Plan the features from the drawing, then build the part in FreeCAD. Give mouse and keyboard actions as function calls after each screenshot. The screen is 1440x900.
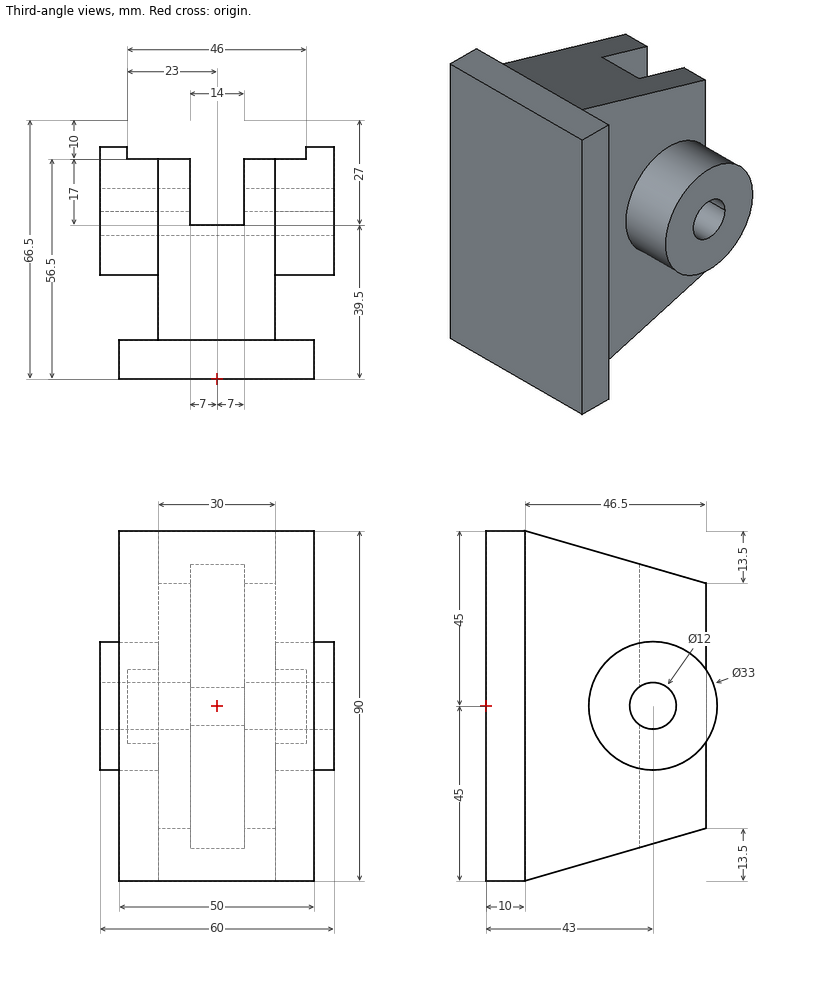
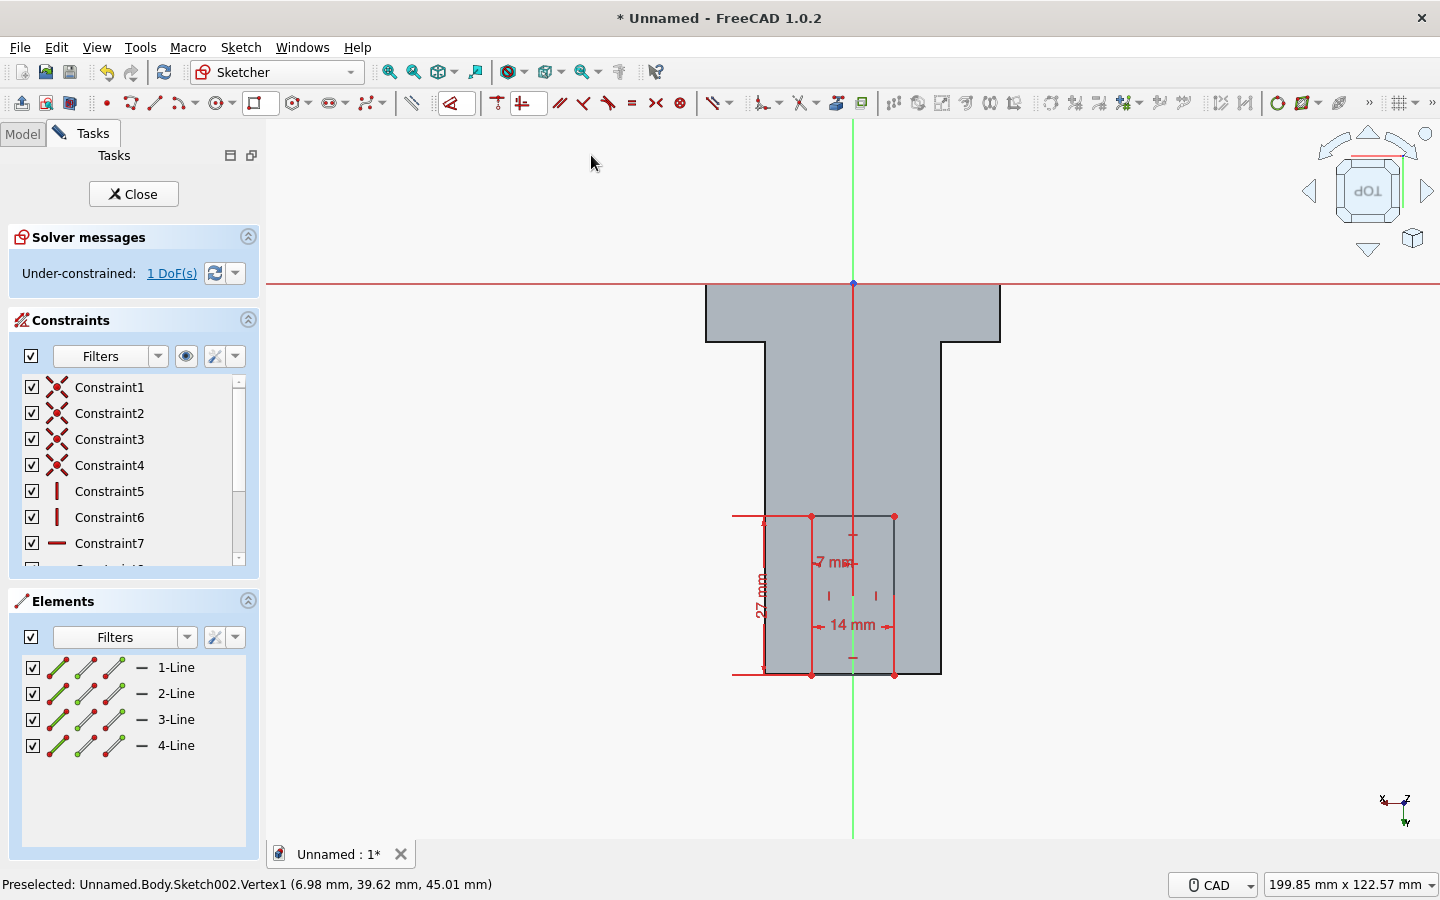
click(812, 516)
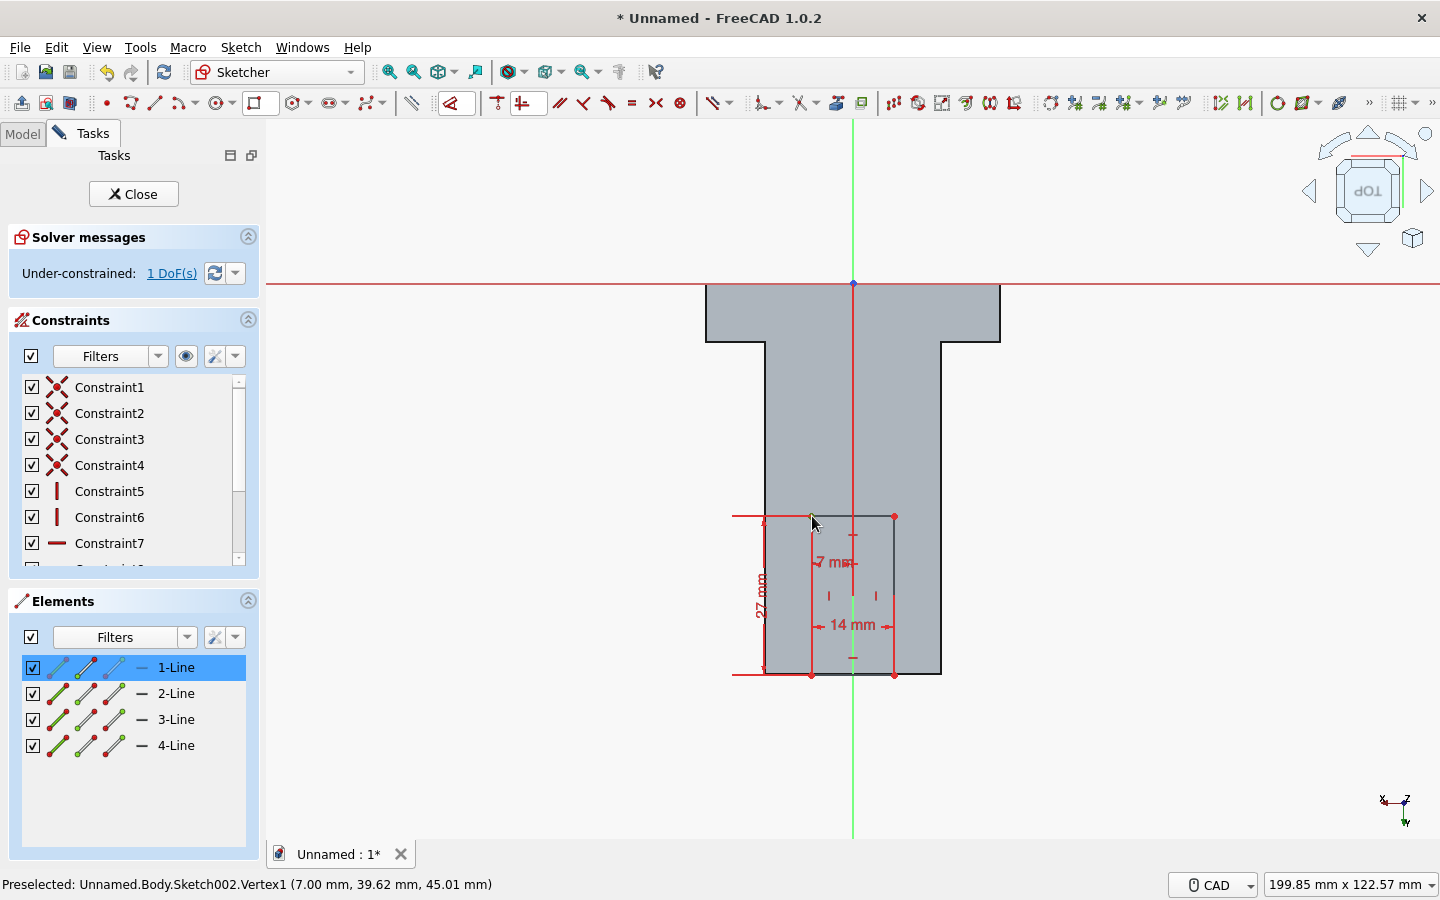
key(i)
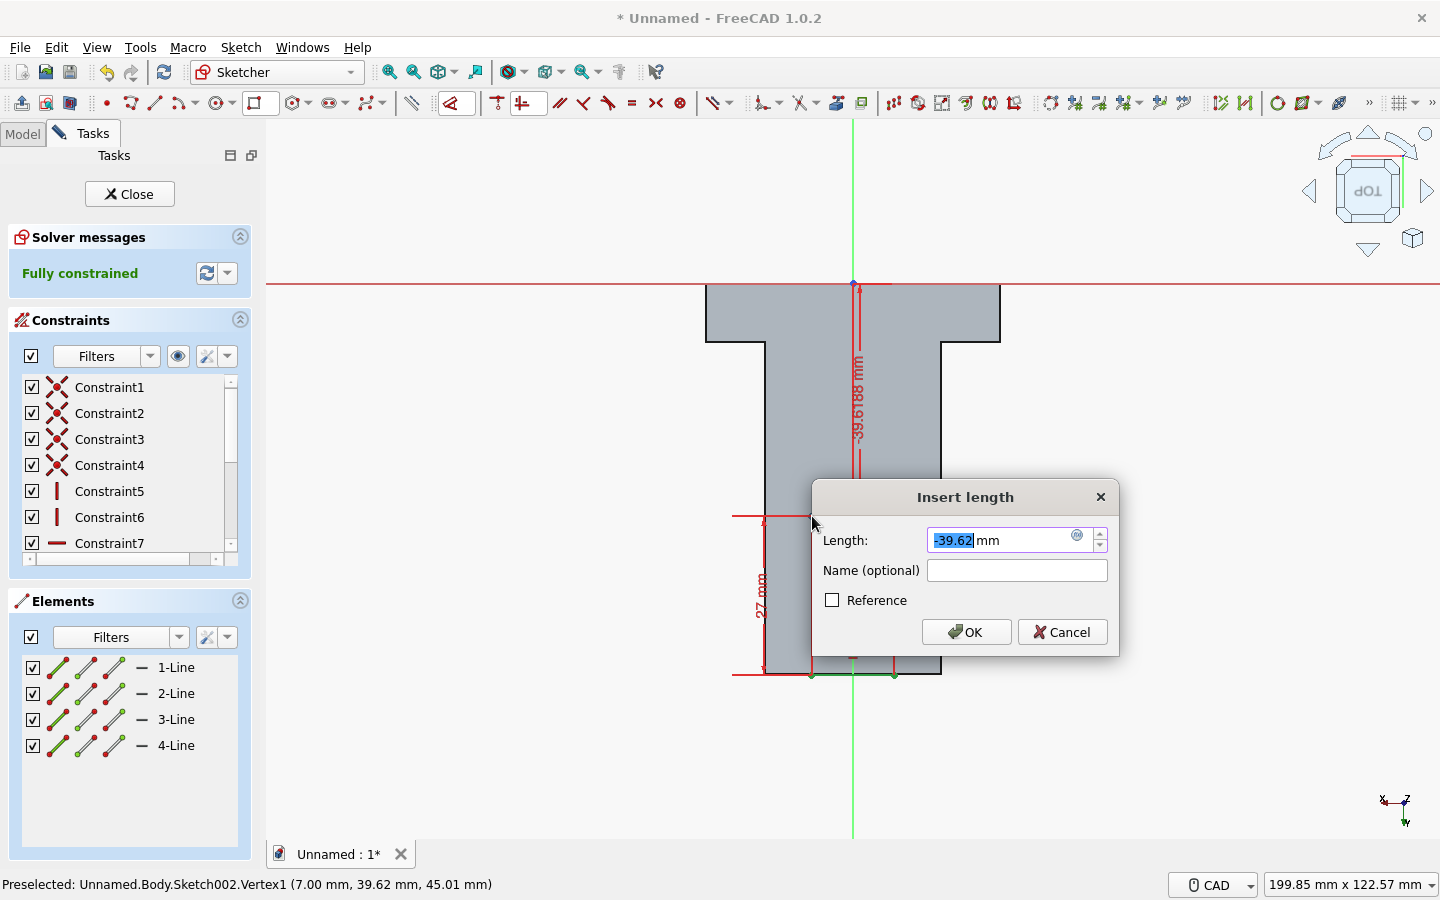
text(-39.5)
key(Return)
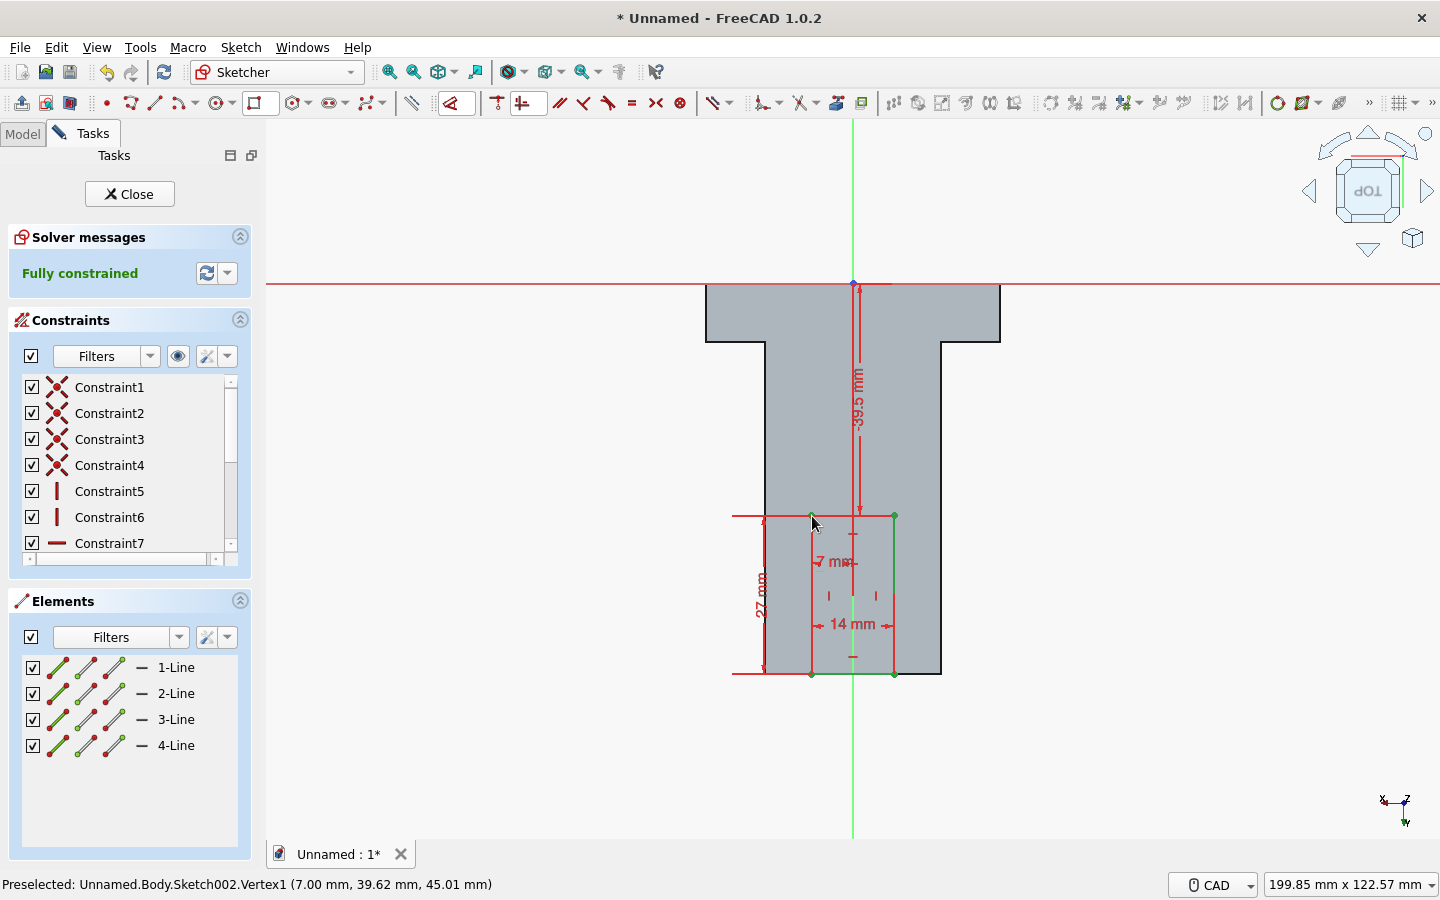
click(130, 194)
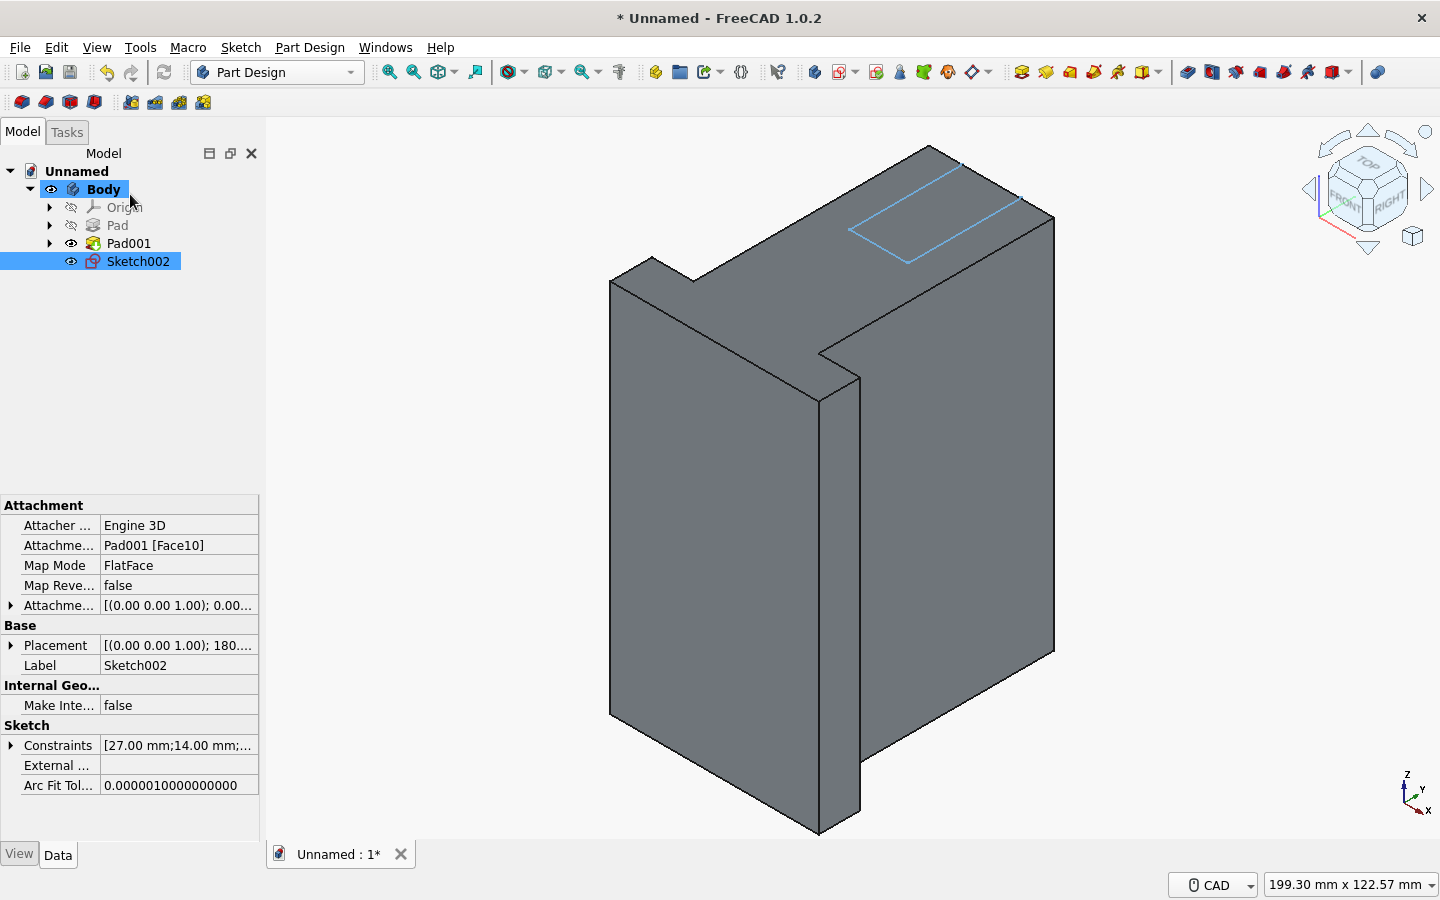
click(1188, 72)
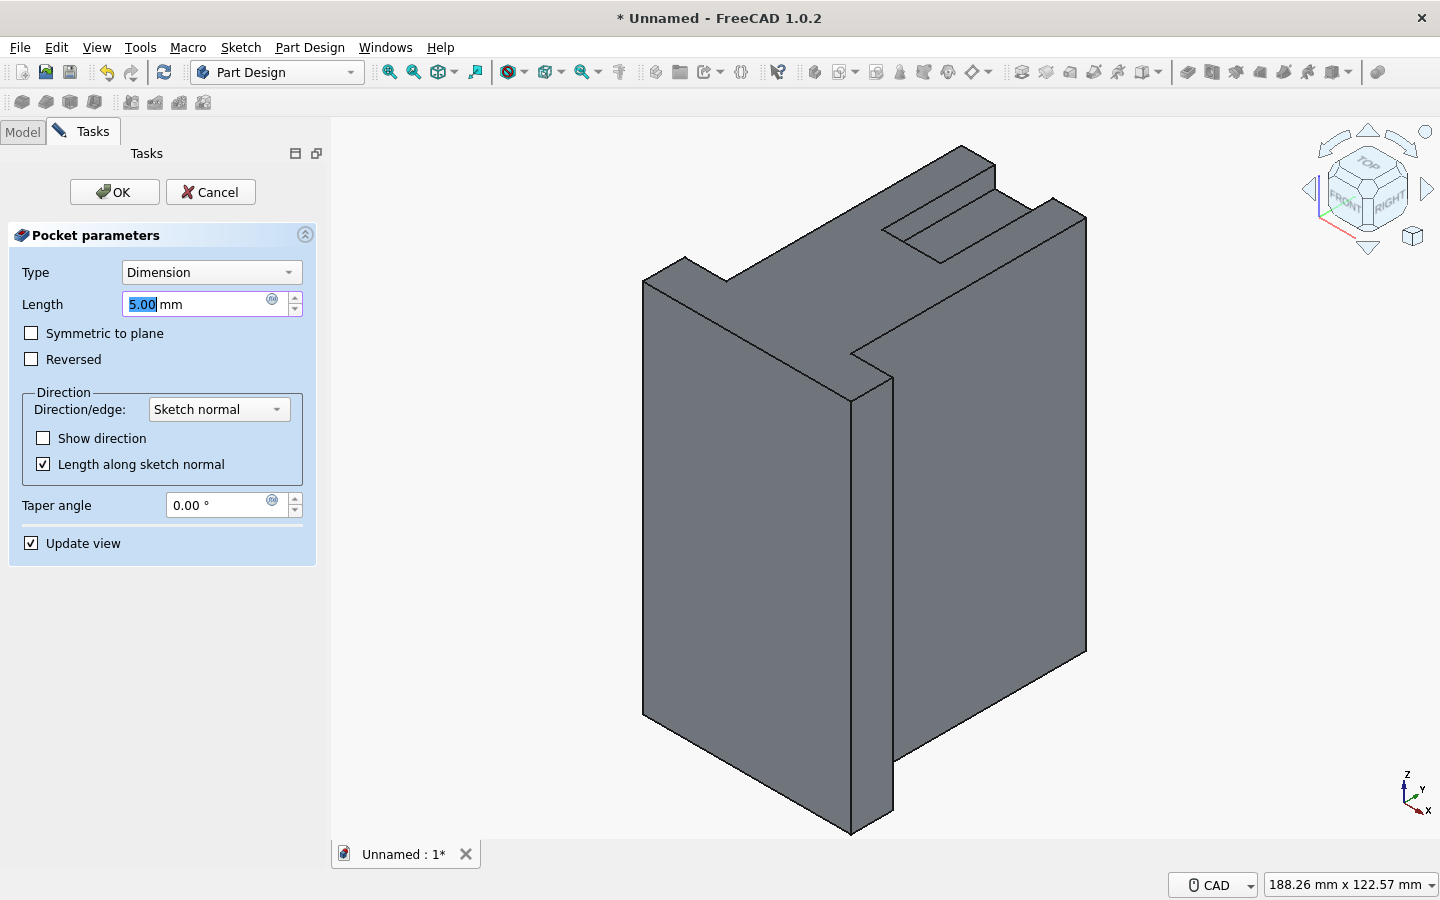
click(212, 272)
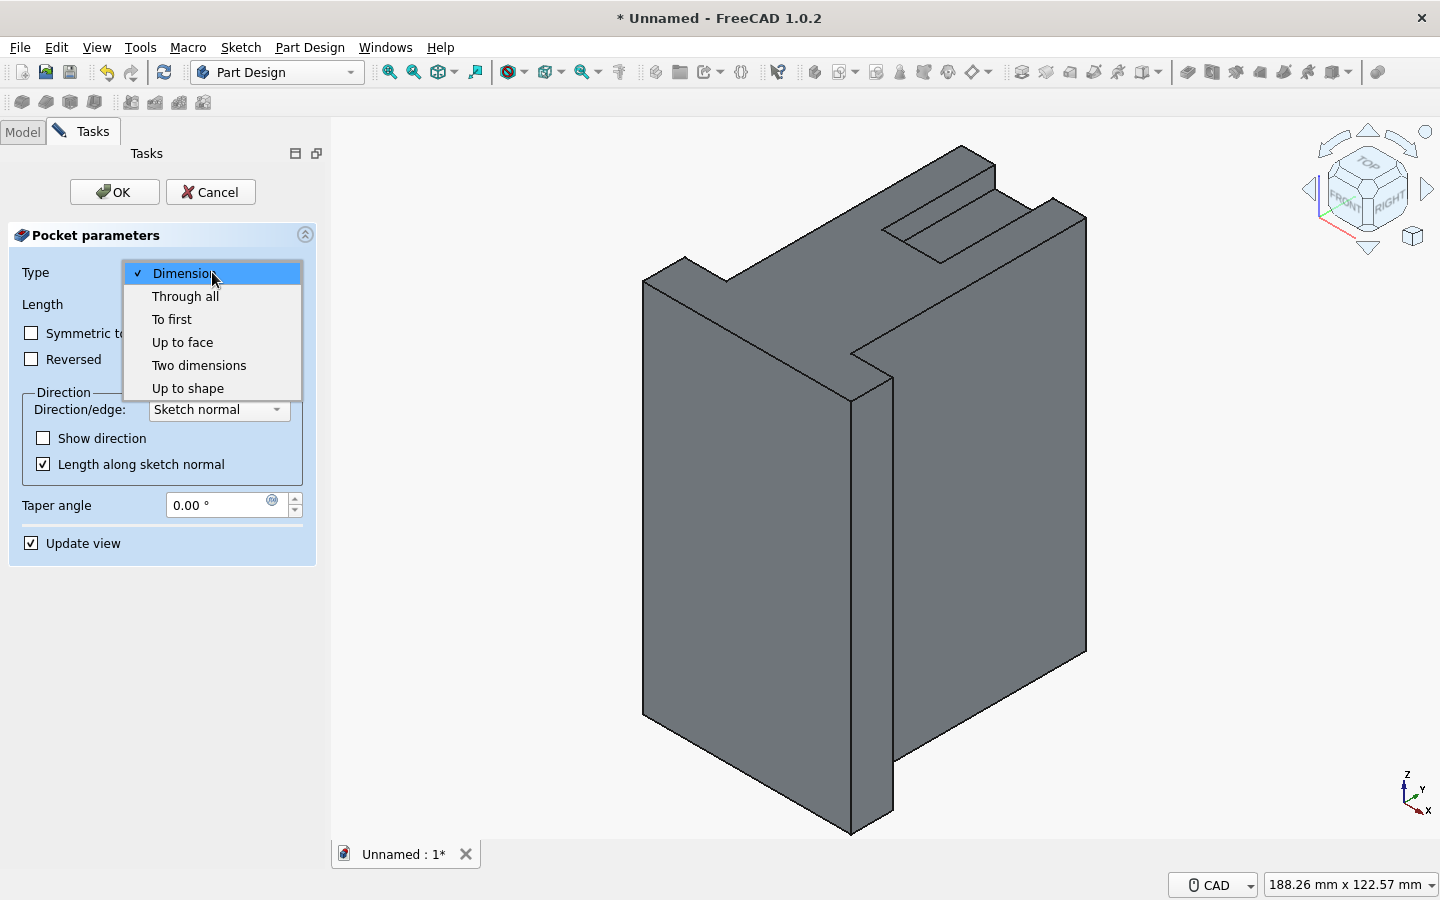
click(212, 296)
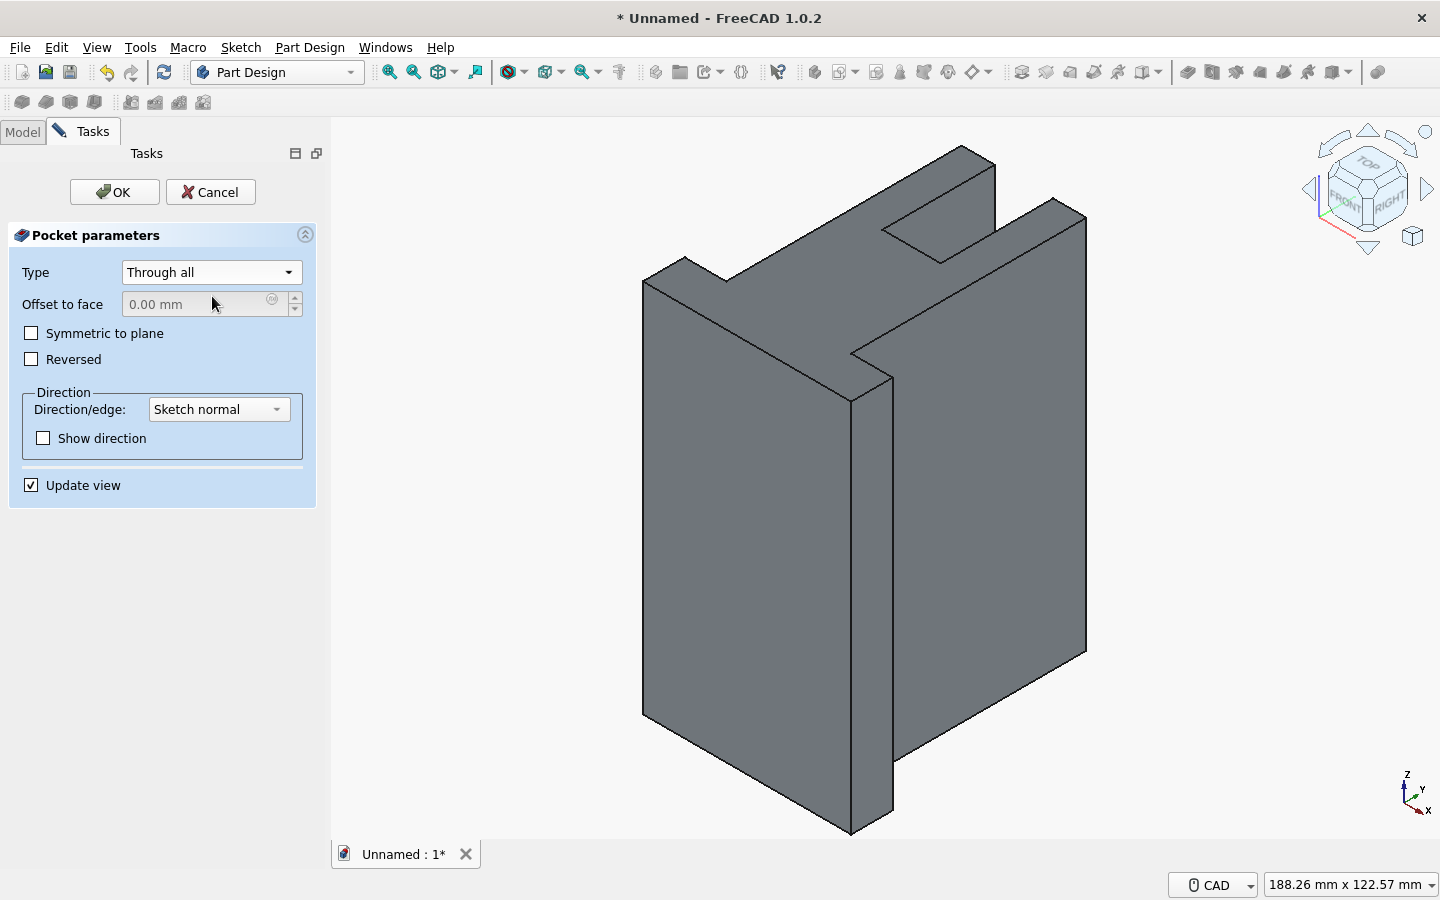
click(115, 192)